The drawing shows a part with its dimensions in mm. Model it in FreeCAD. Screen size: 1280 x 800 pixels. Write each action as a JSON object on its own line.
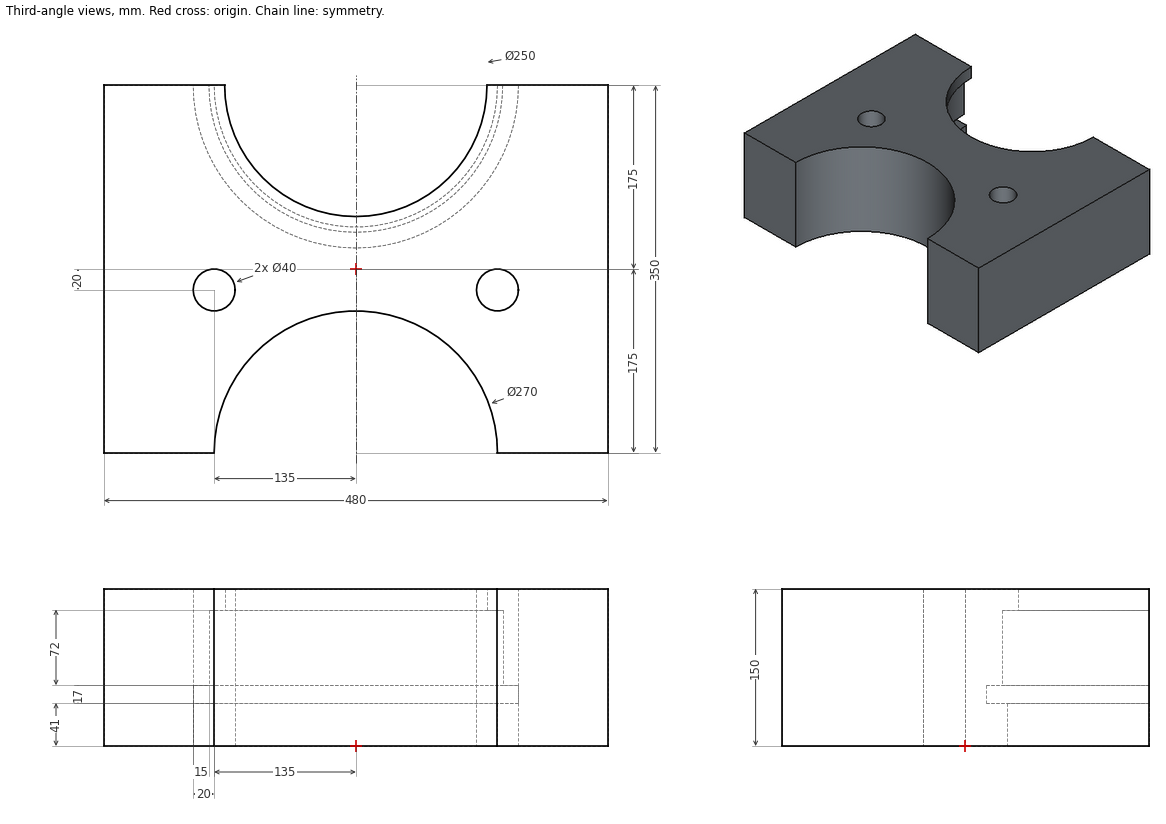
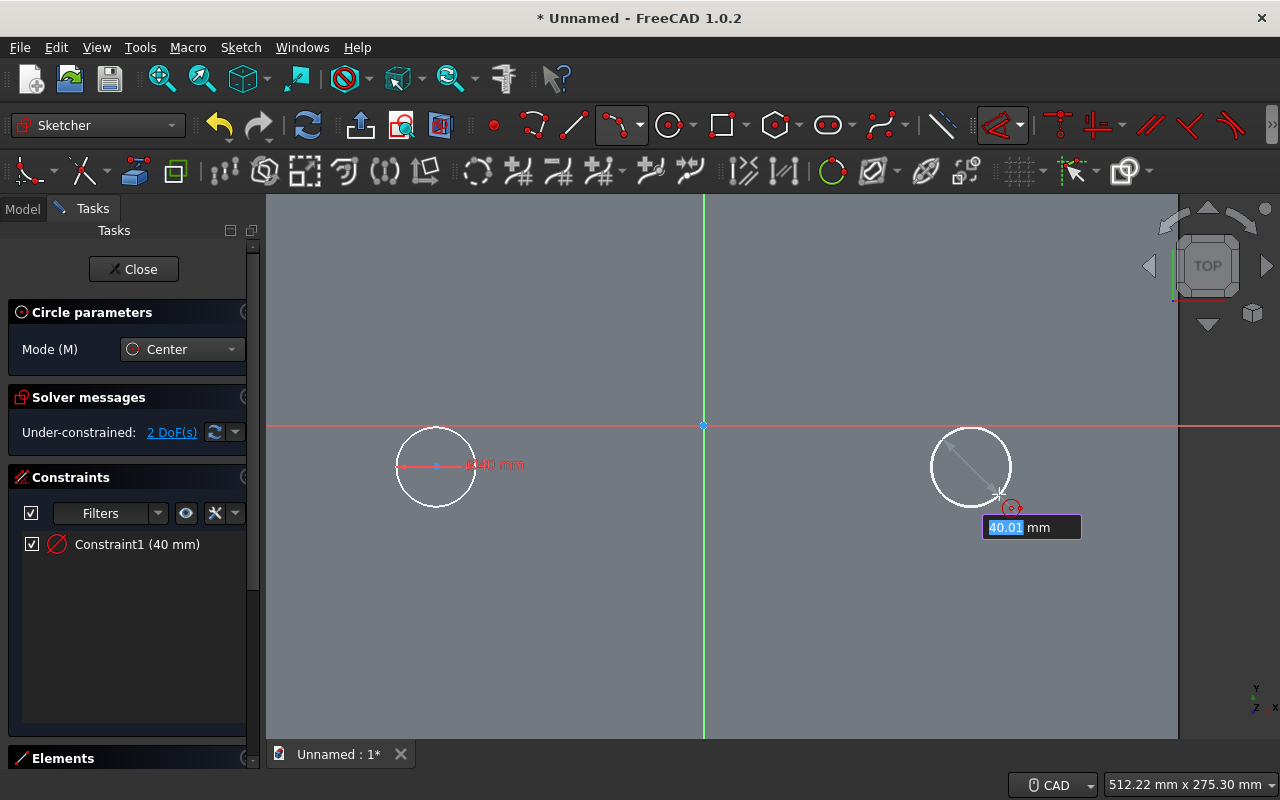
{"action": "type", "text": "40"}
{"action": "key", "text": "Return"}
{"action": "key", "text": "Escape"}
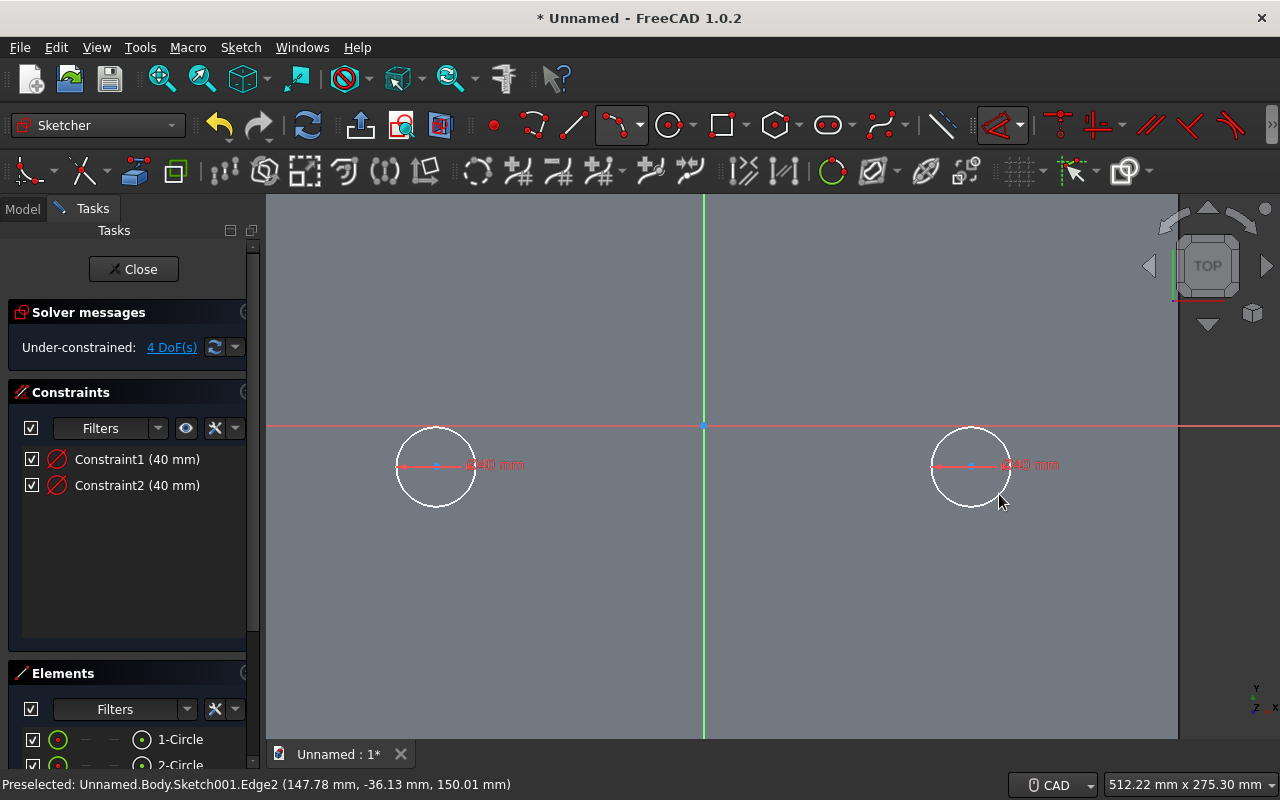
{"action": "left_click", "coordinate": [436, 467]}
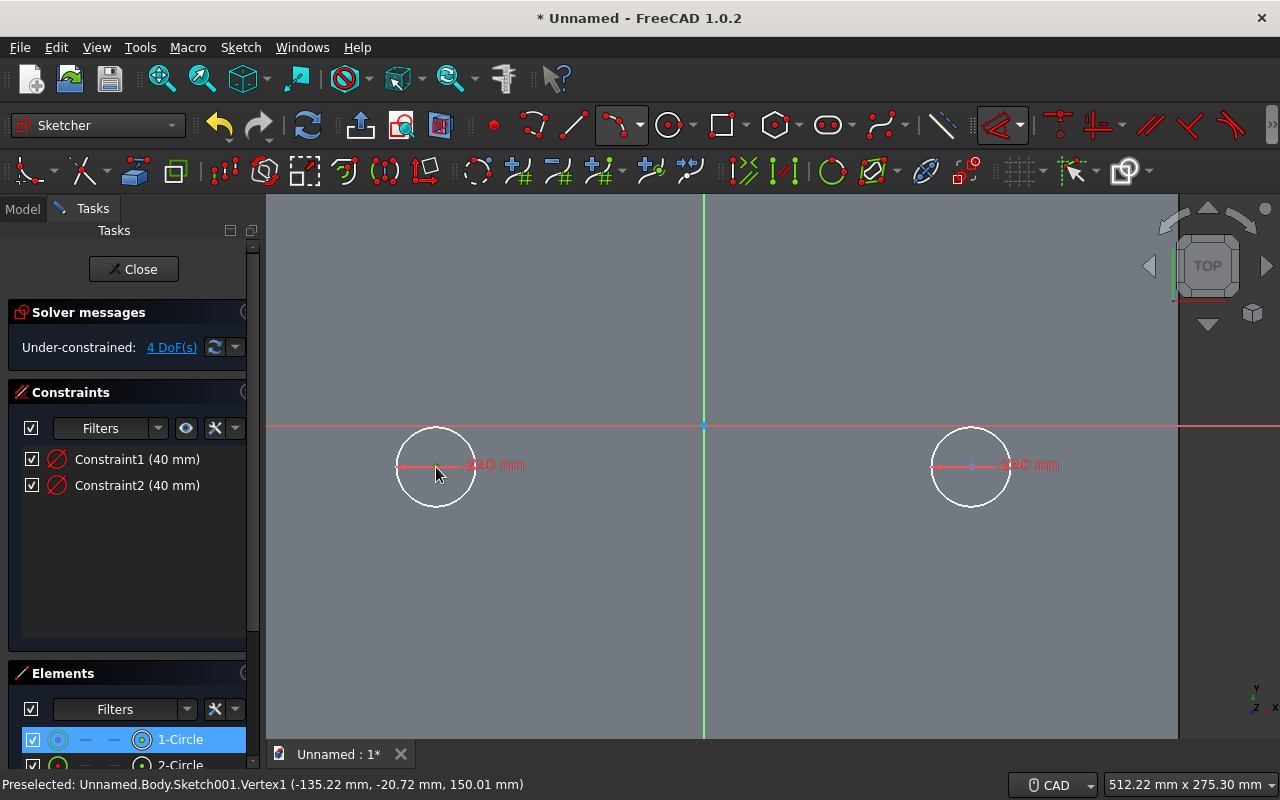
{"action": "left_click", "coordinate": [971, 467]}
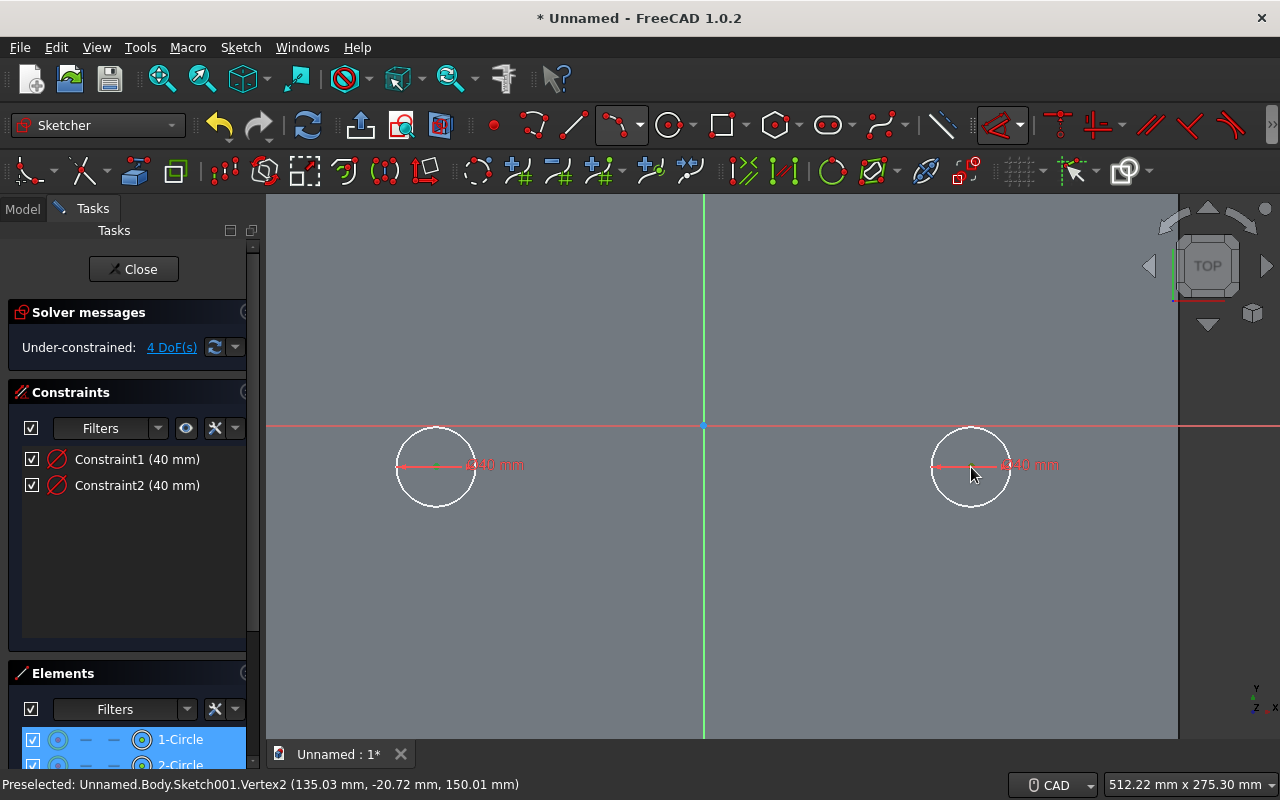
{"action": "left_click", "coordinate": [704, 676]}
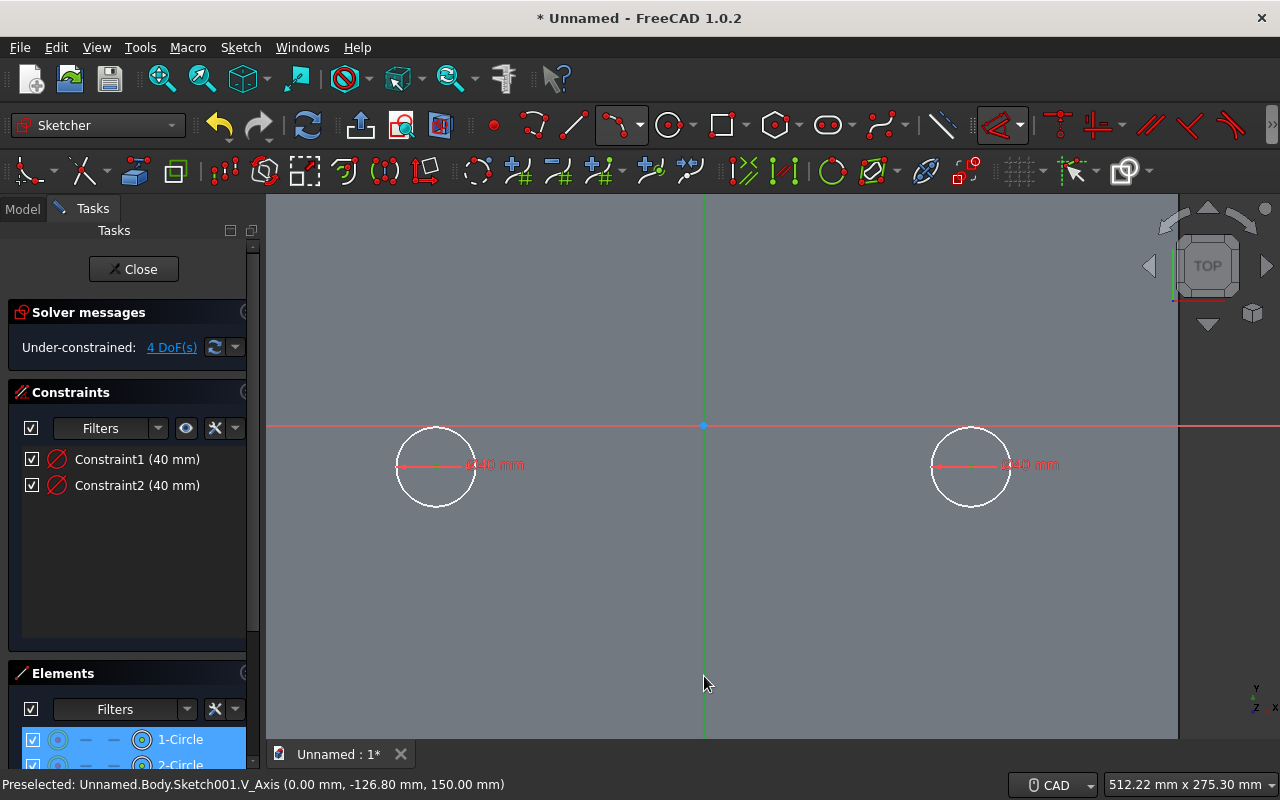
{"action": "key", "text": "s"}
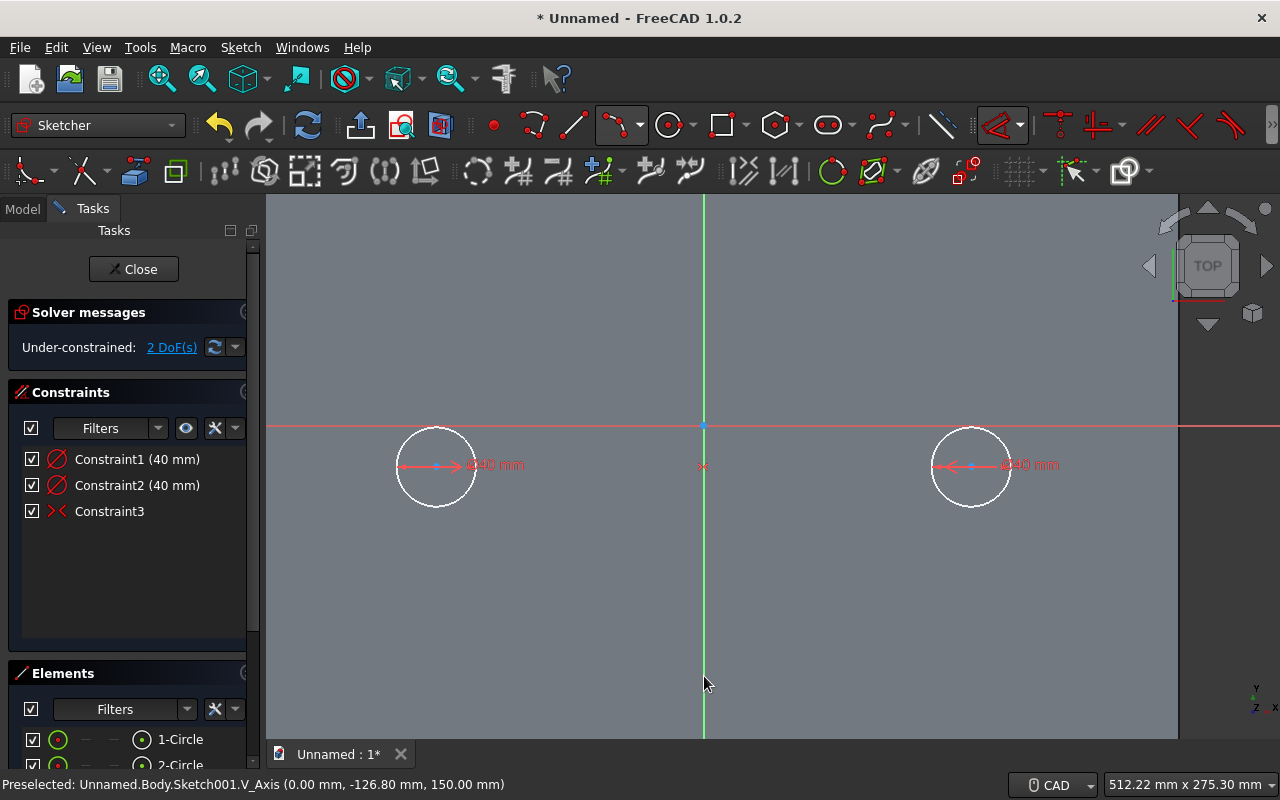
{"action": "left_click", "coordinate": [996, 126]}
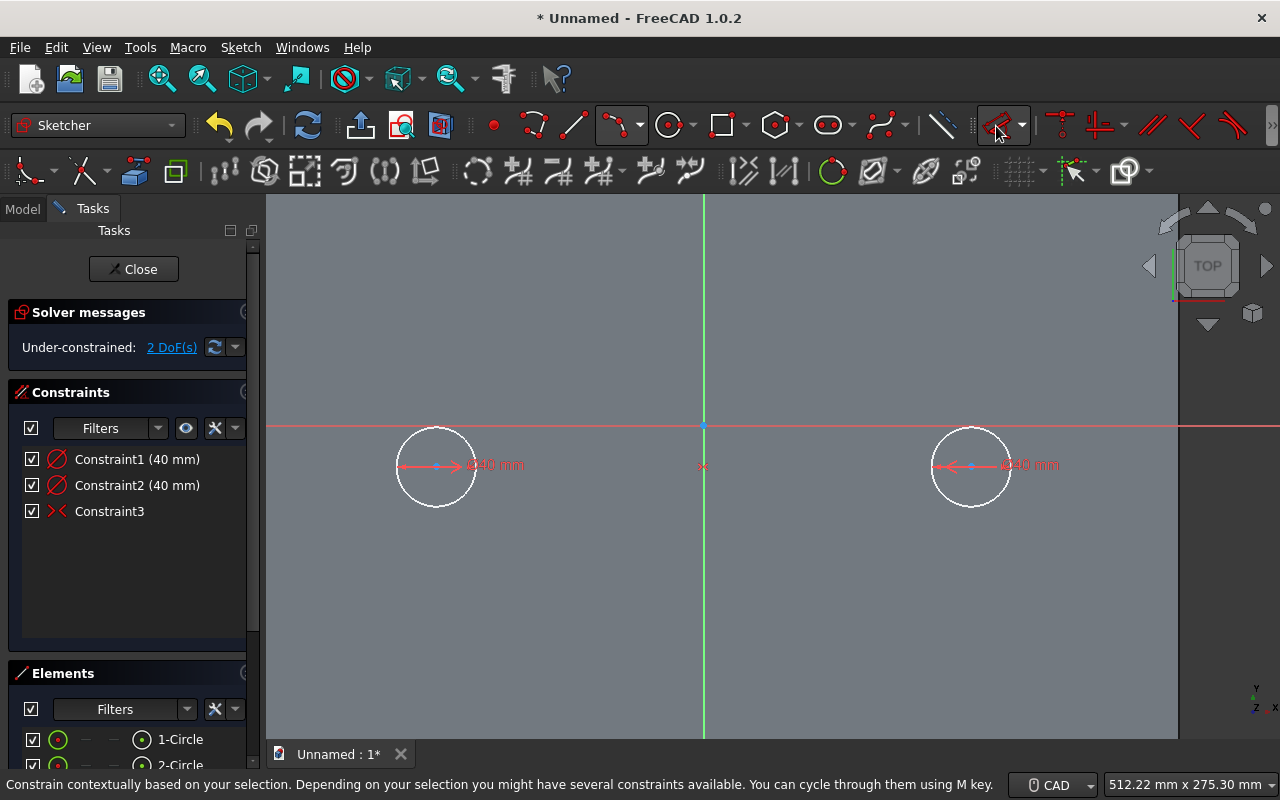
{"action": "left_click", "coordinate": [436, 467]}
{"action": "left_click", "coordinate": [738, 446]}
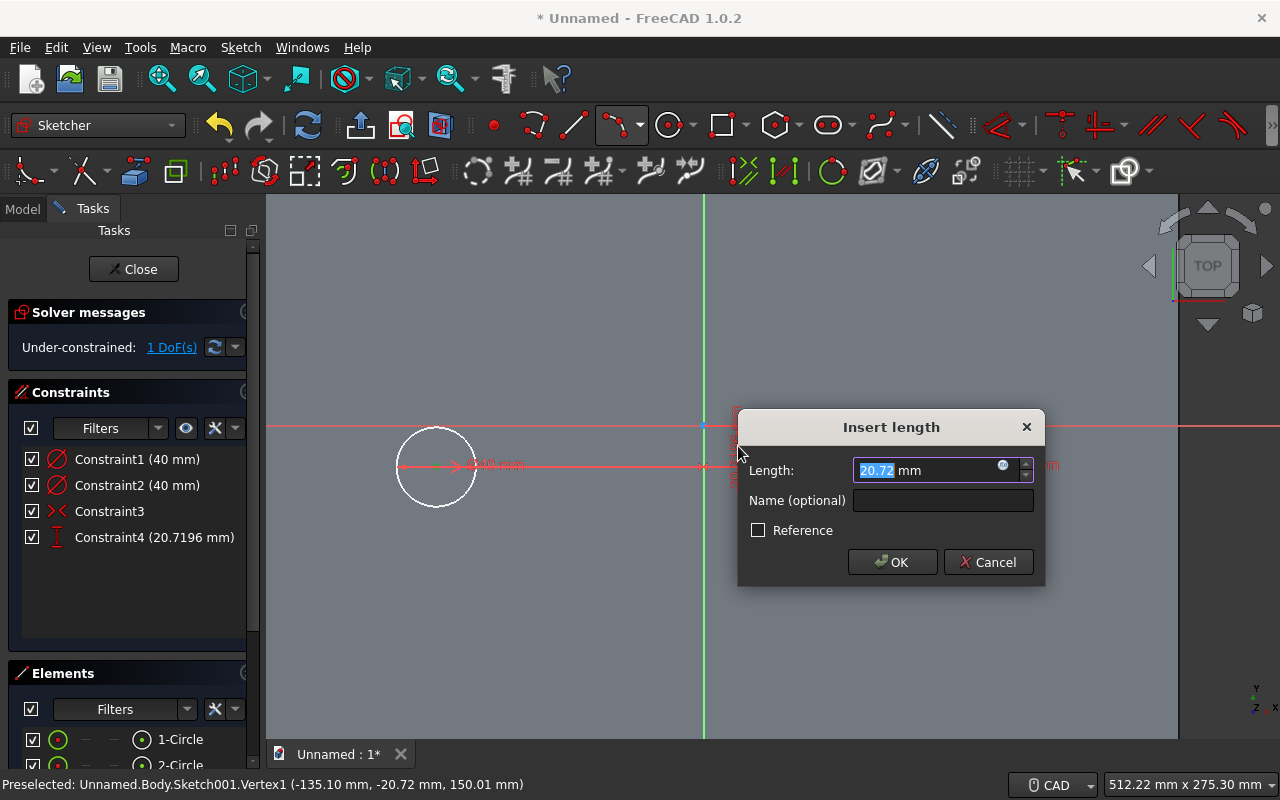
{"action": "type", "text": "20"}
{"action": "key", "text": "Return"}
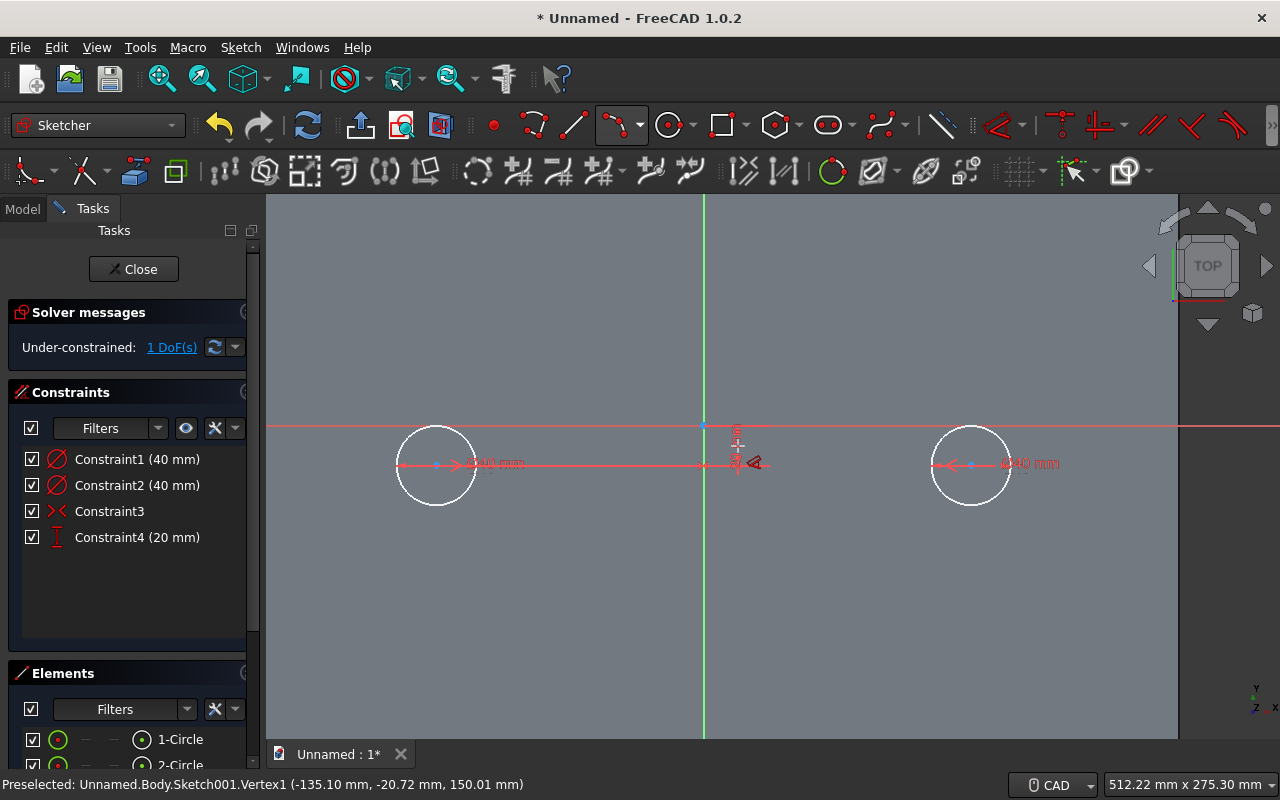
{"action": "left_click", "coordinate": [436, 466]}
{"action": "left_click", "coordinate": [570, 392]}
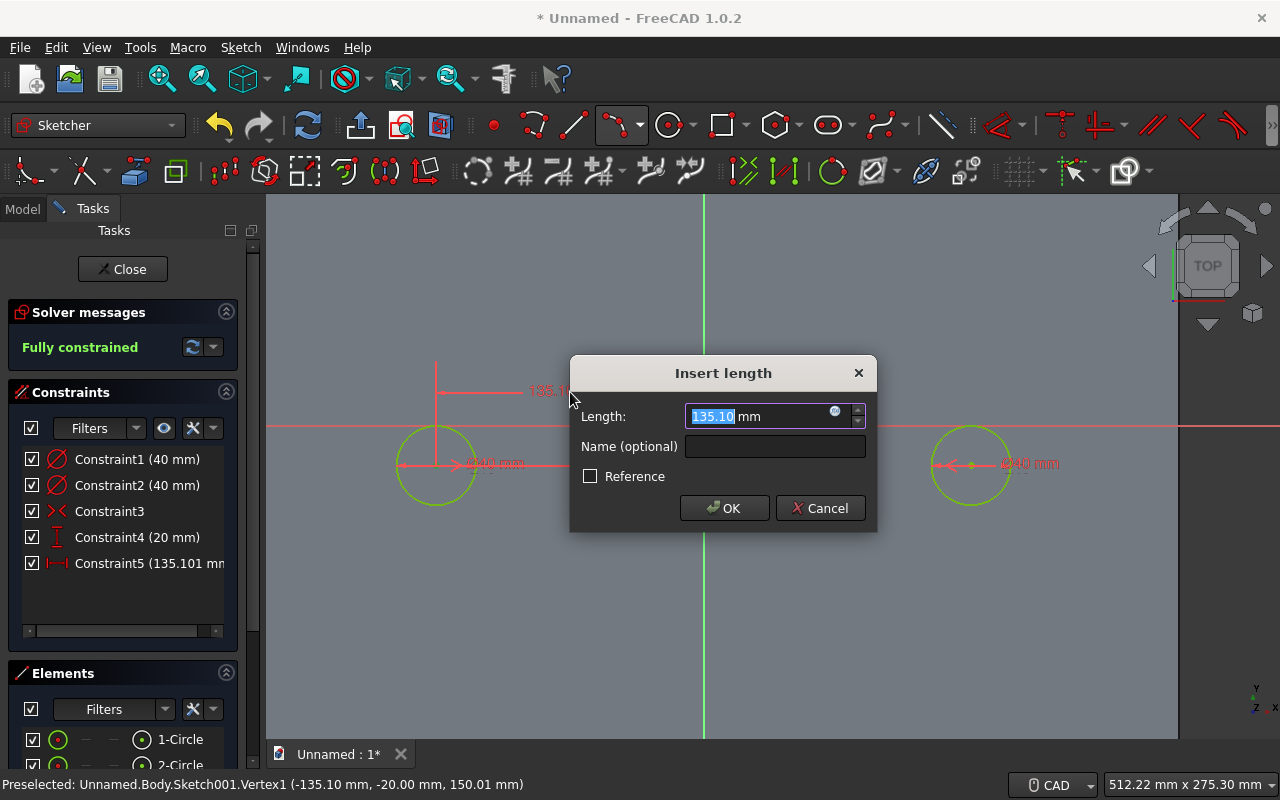
{"action": "type", "text": "135"}
{"action": "key", "text": "Return"}
{"action": "key", "text": "Escape"}